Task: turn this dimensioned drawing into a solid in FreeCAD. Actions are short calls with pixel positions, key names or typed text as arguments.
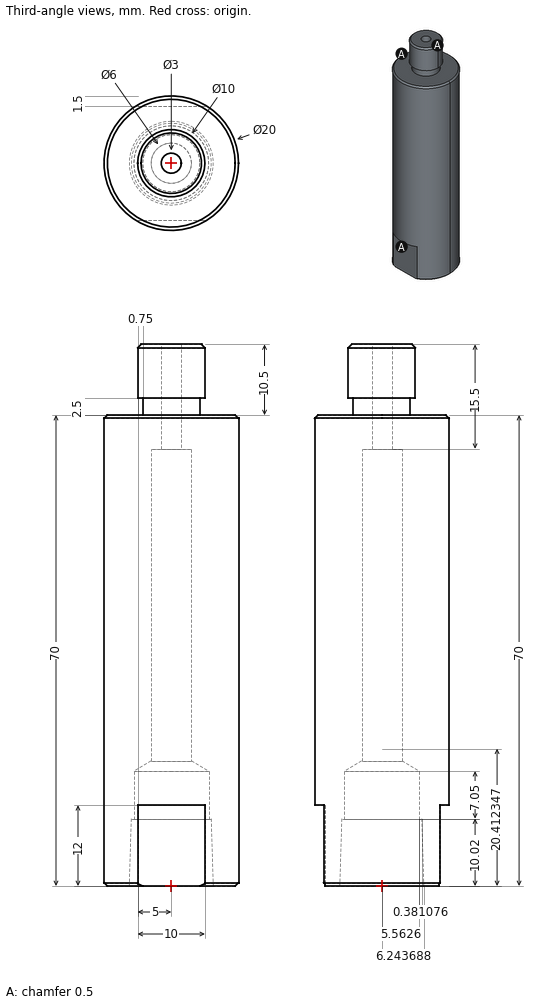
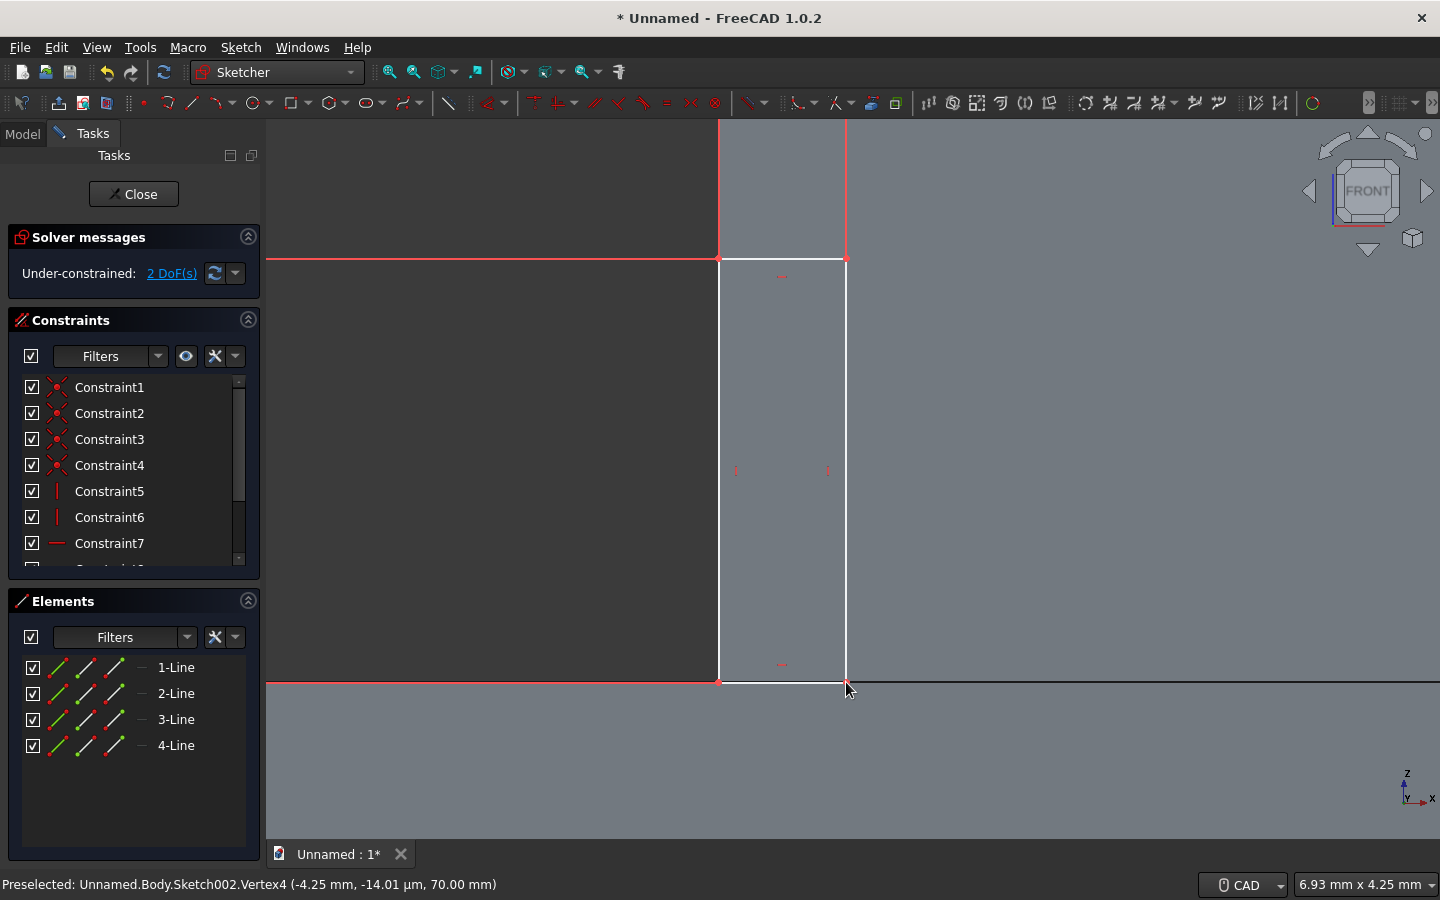
key(d)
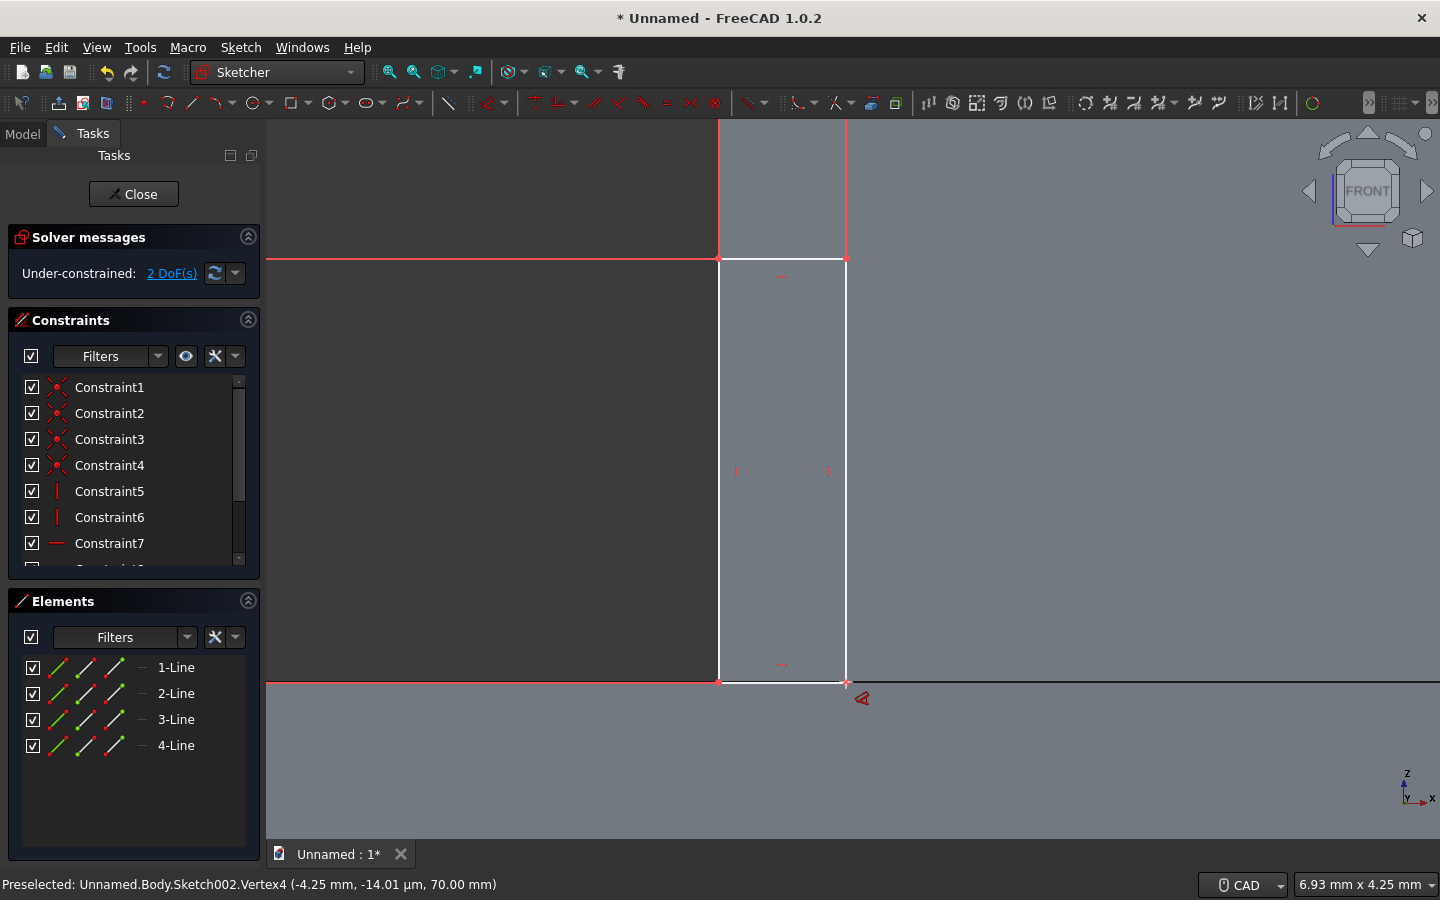
click(719, 259)
click(997, 225)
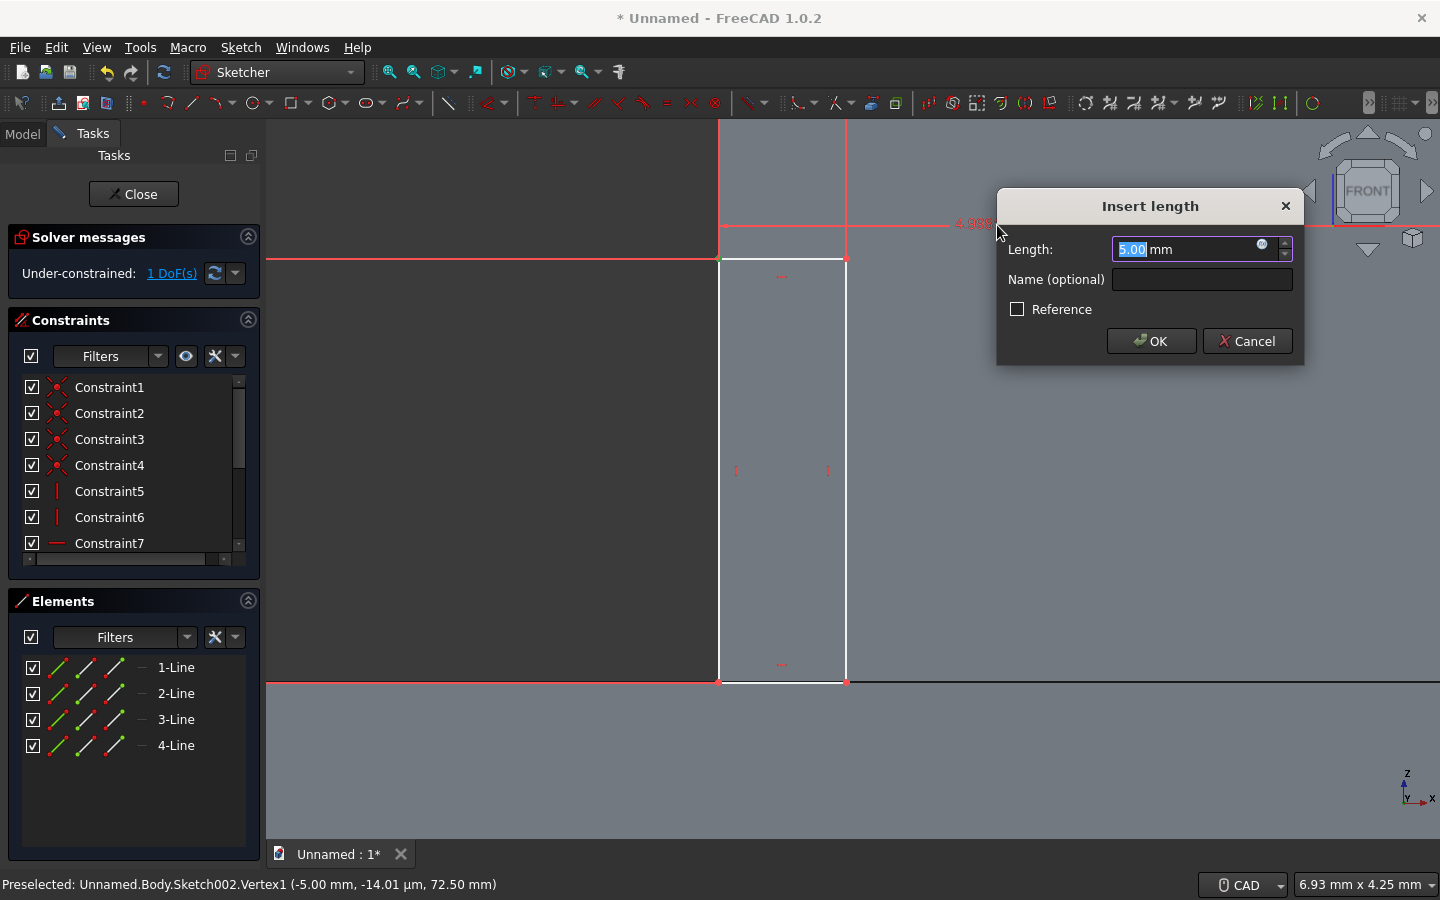
text(5)
key(Return)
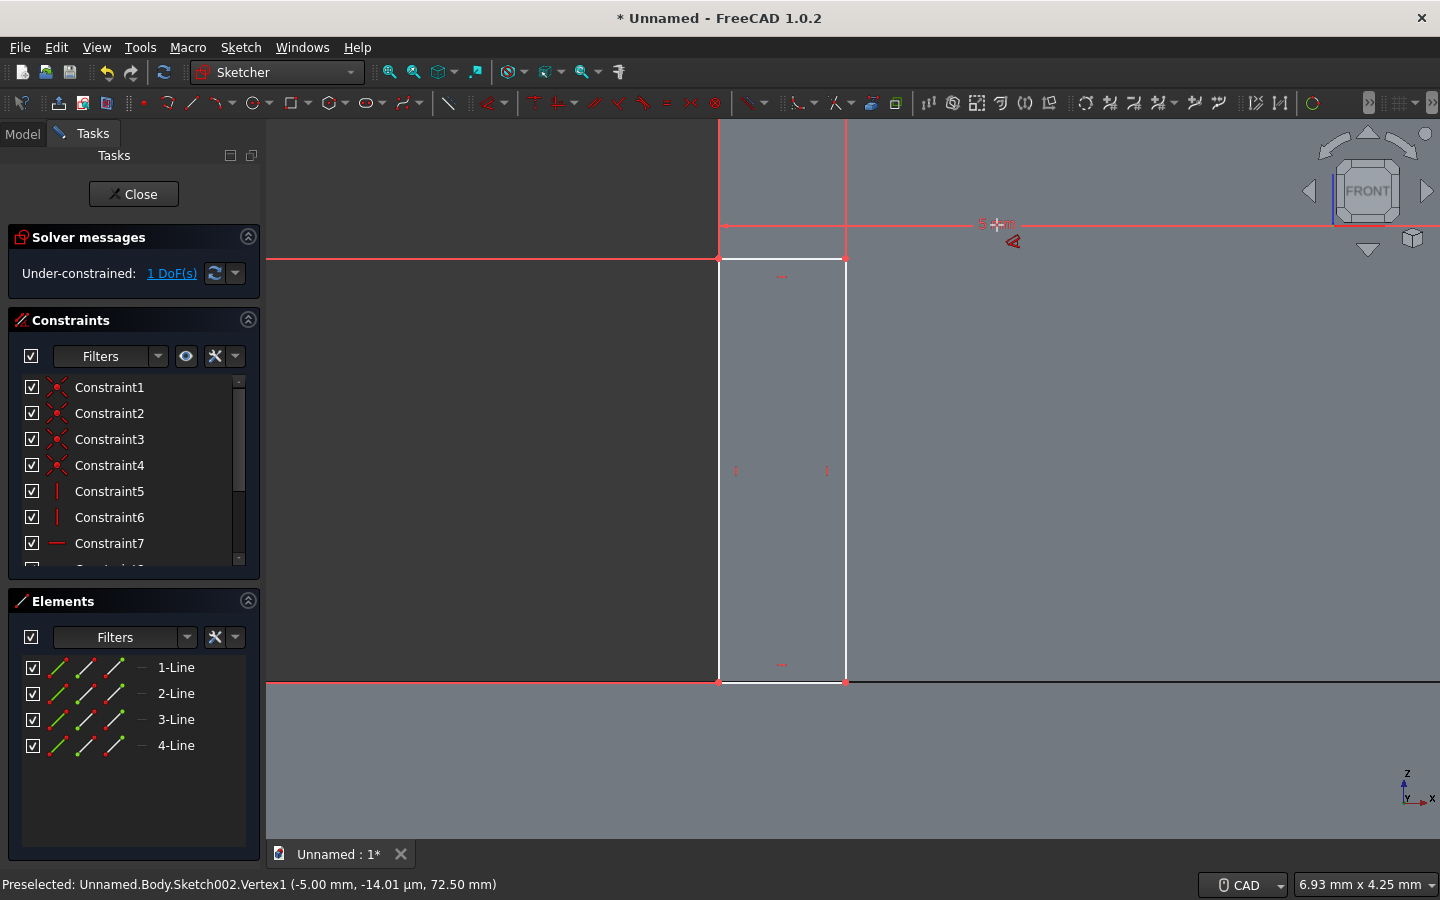
click(719, 683)
click(685, 747)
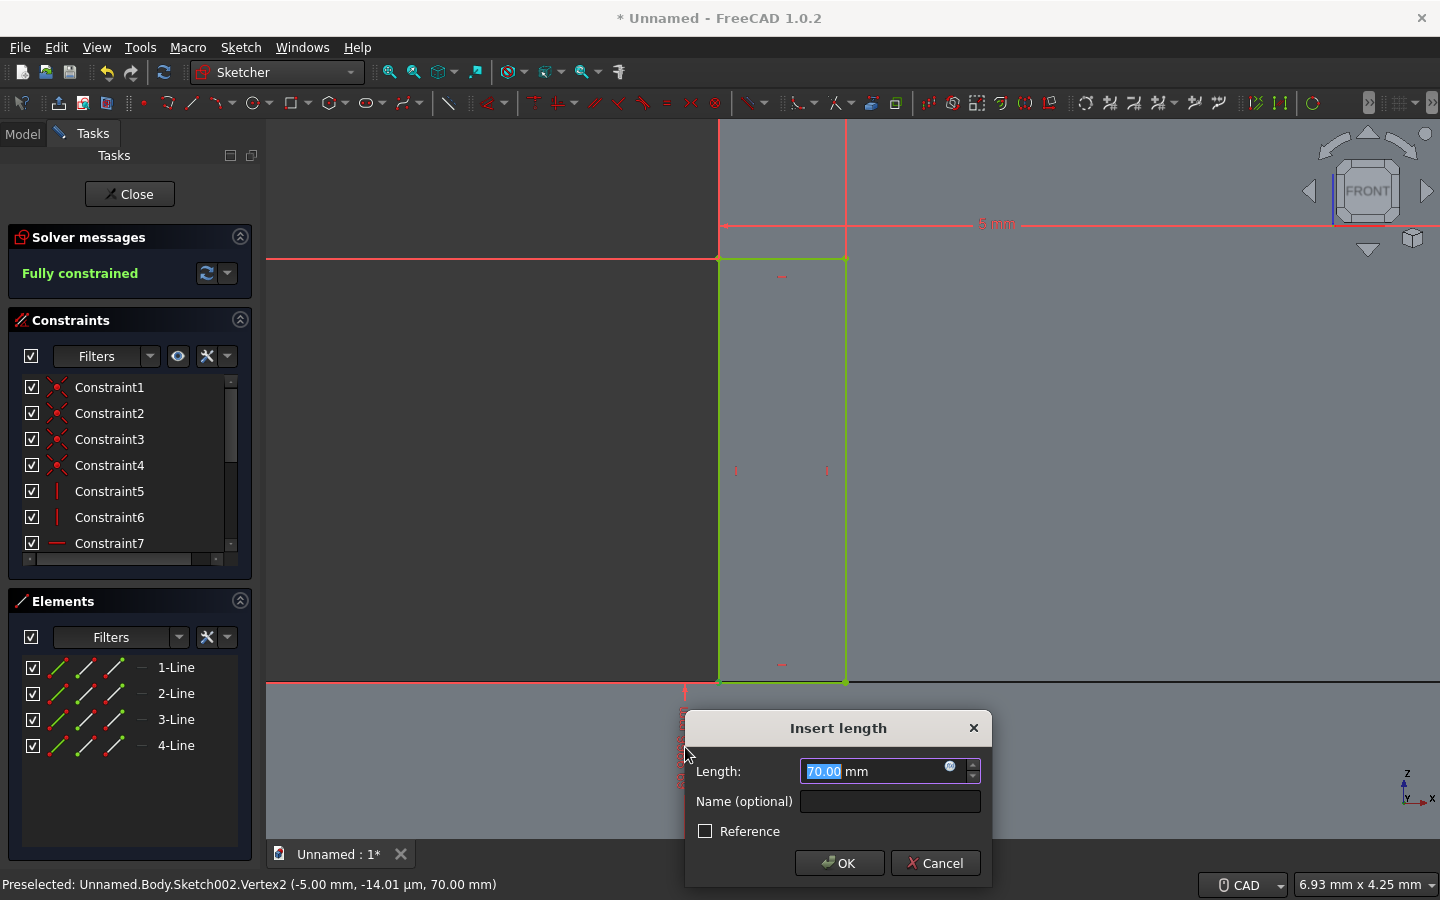
text(70)
key(Return)
key(Escape)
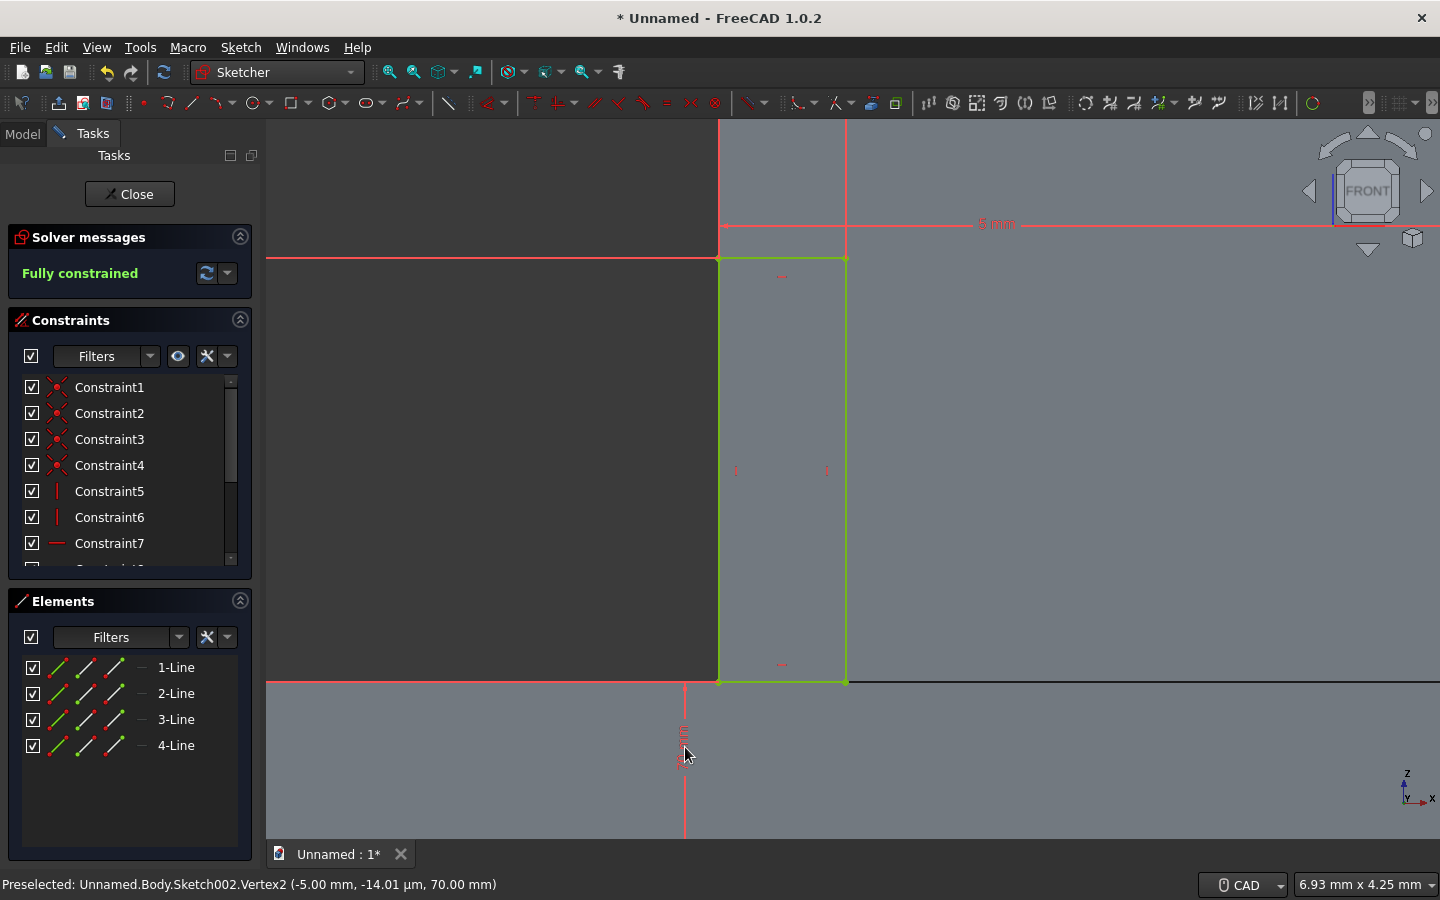
click(130, 194)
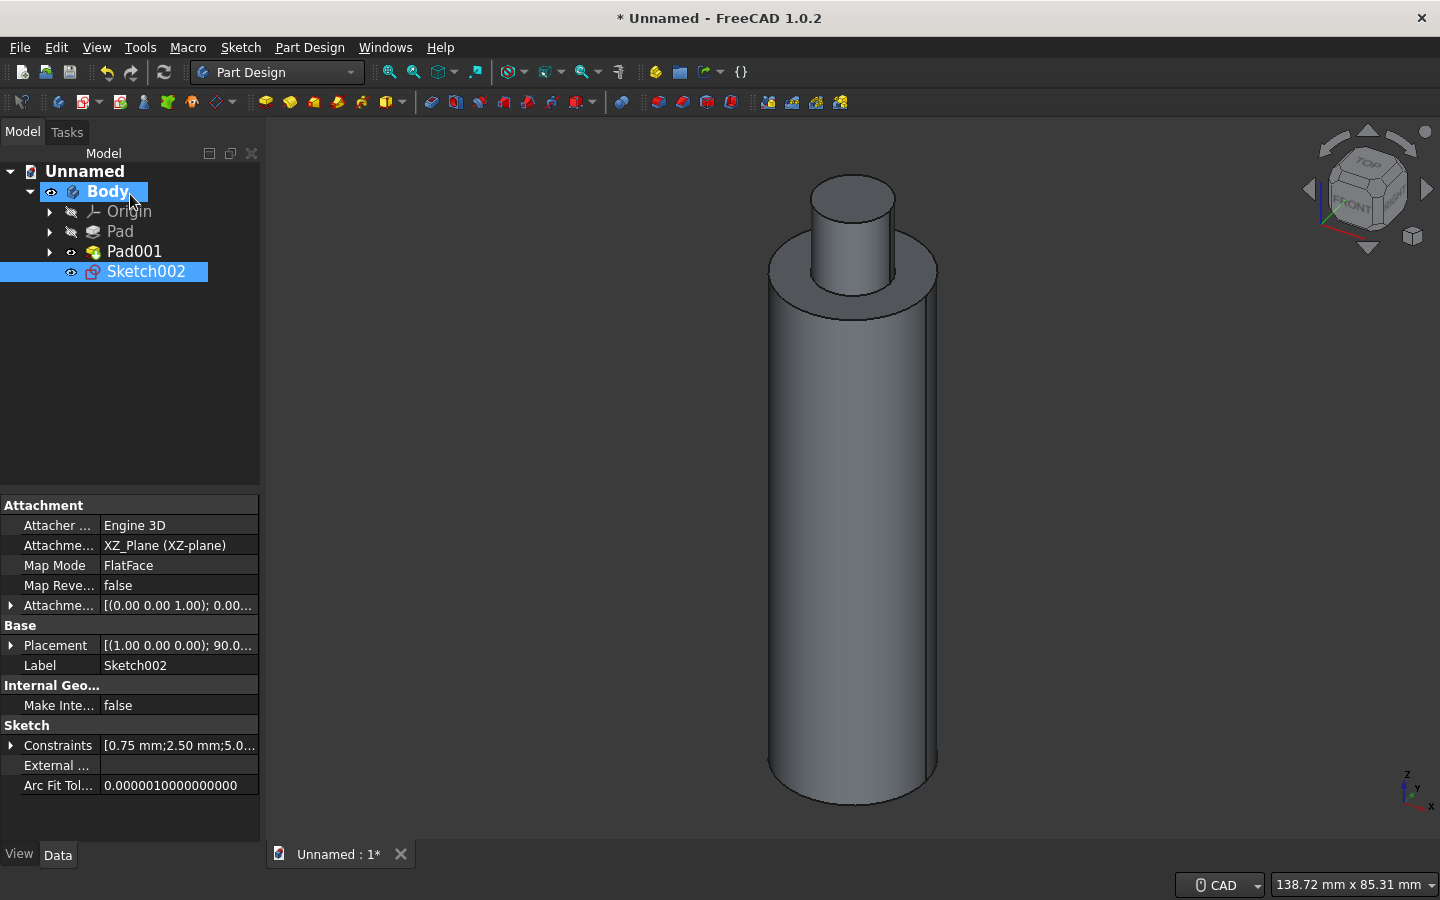
click(480, 102)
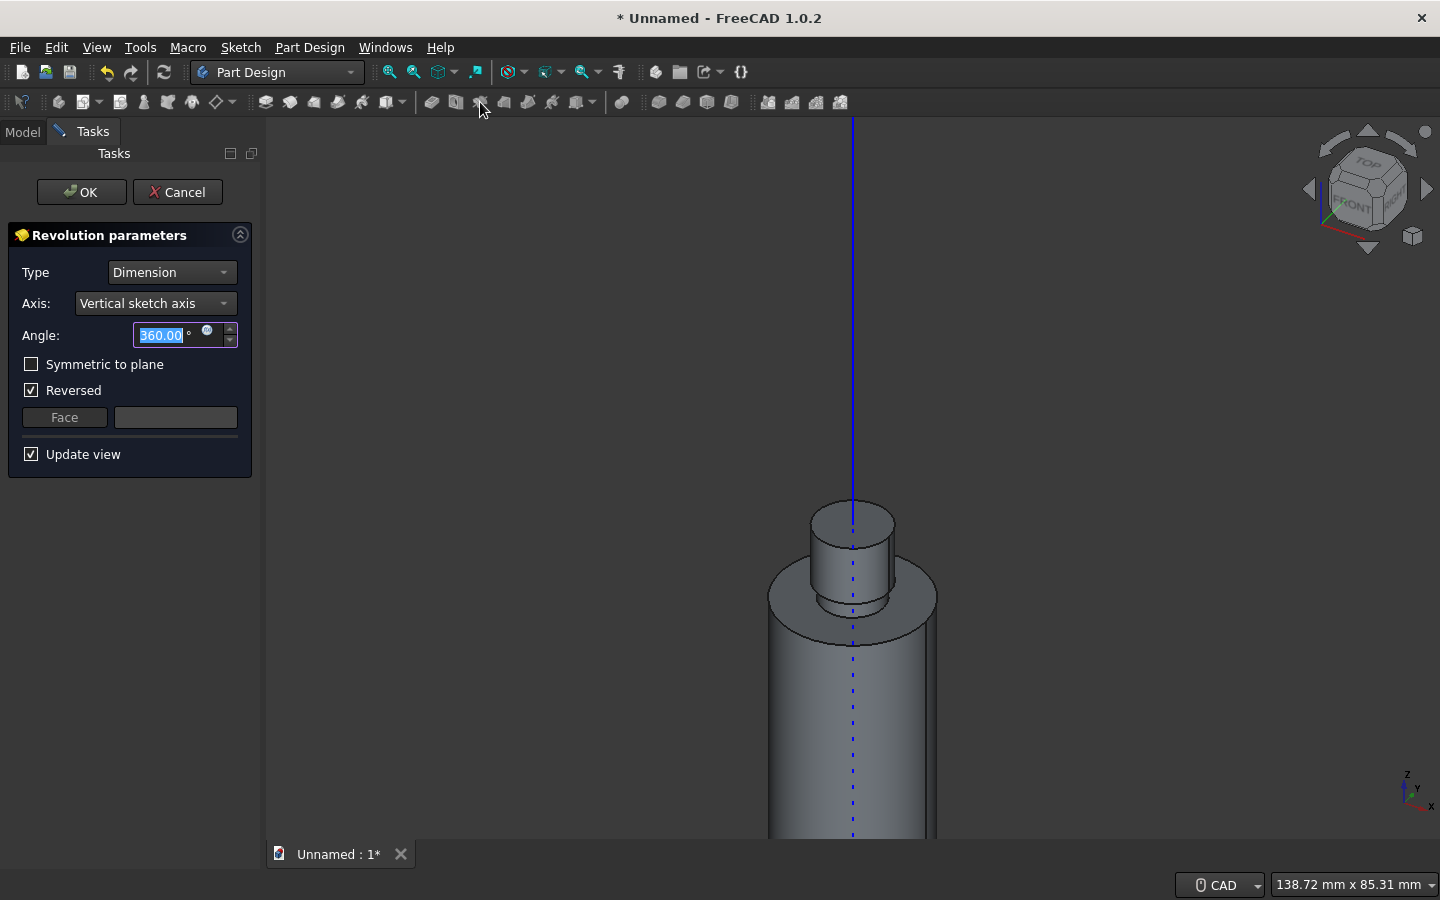
click(82, 192)